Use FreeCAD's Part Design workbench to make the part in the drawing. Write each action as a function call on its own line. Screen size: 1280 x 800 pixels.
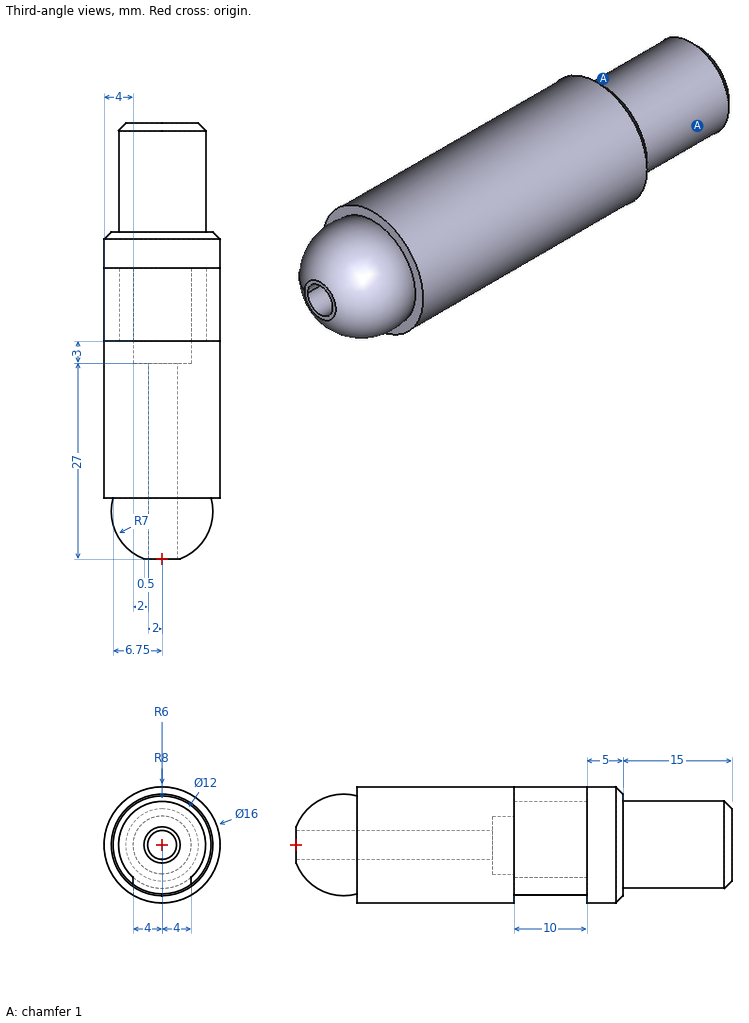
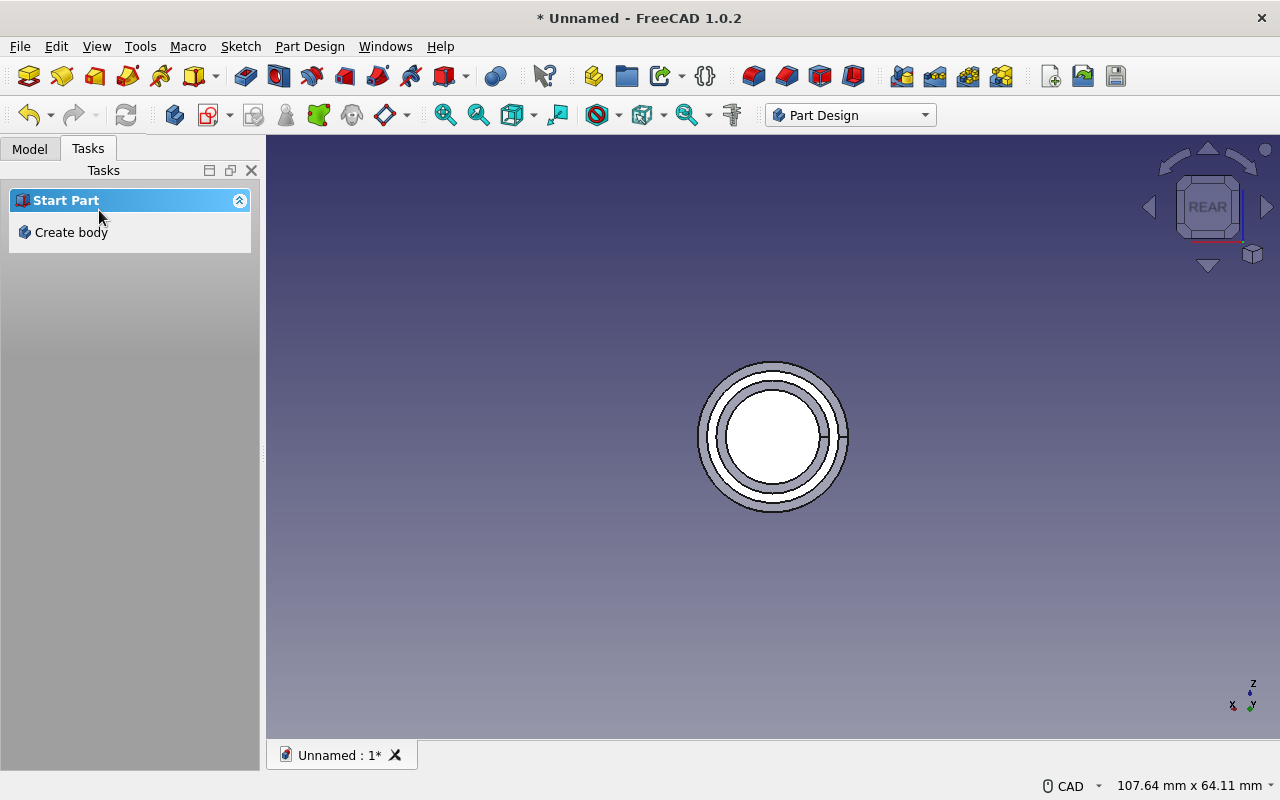
key(0)